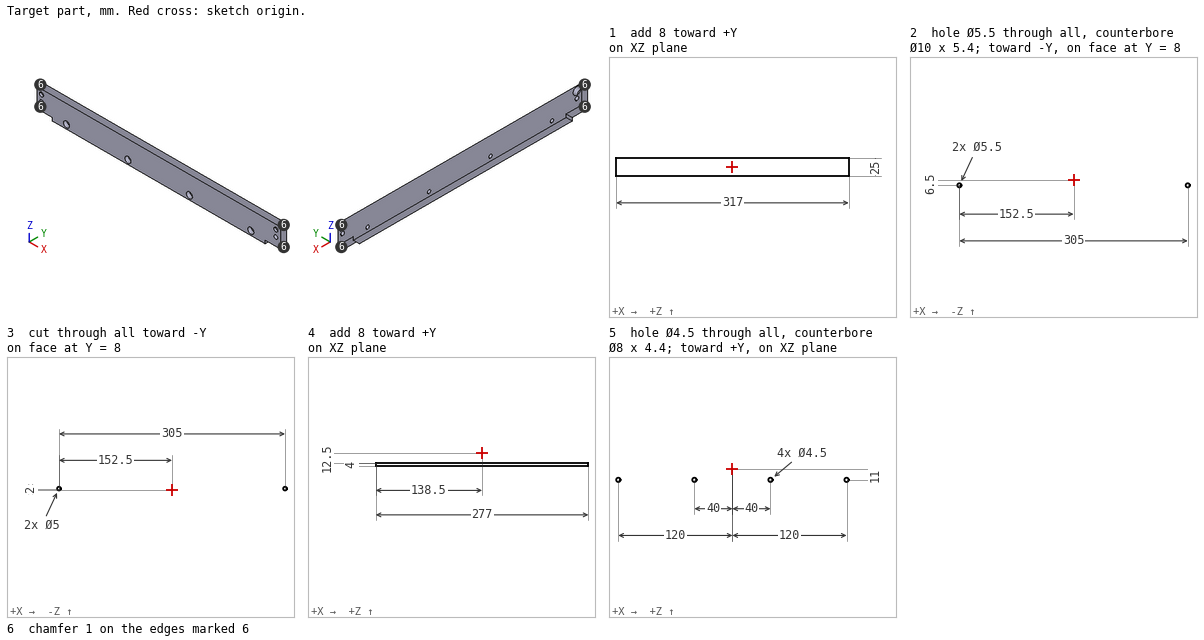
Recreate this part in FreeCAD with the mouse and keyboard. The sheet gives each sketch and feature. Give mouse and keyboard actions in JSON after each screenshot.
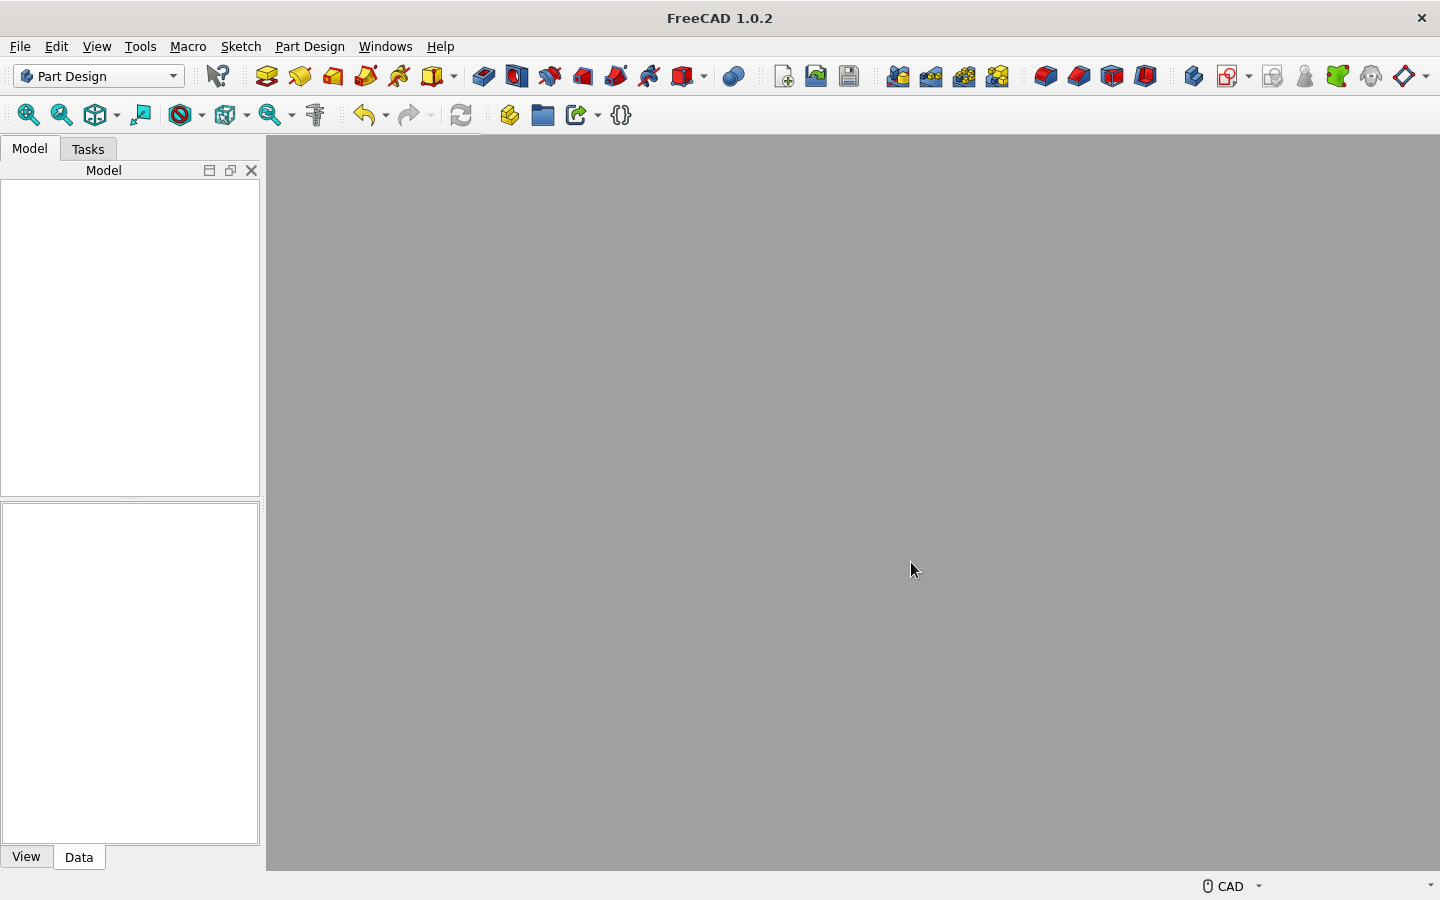
{"action": "left_click", "coordinate": [783, 76]}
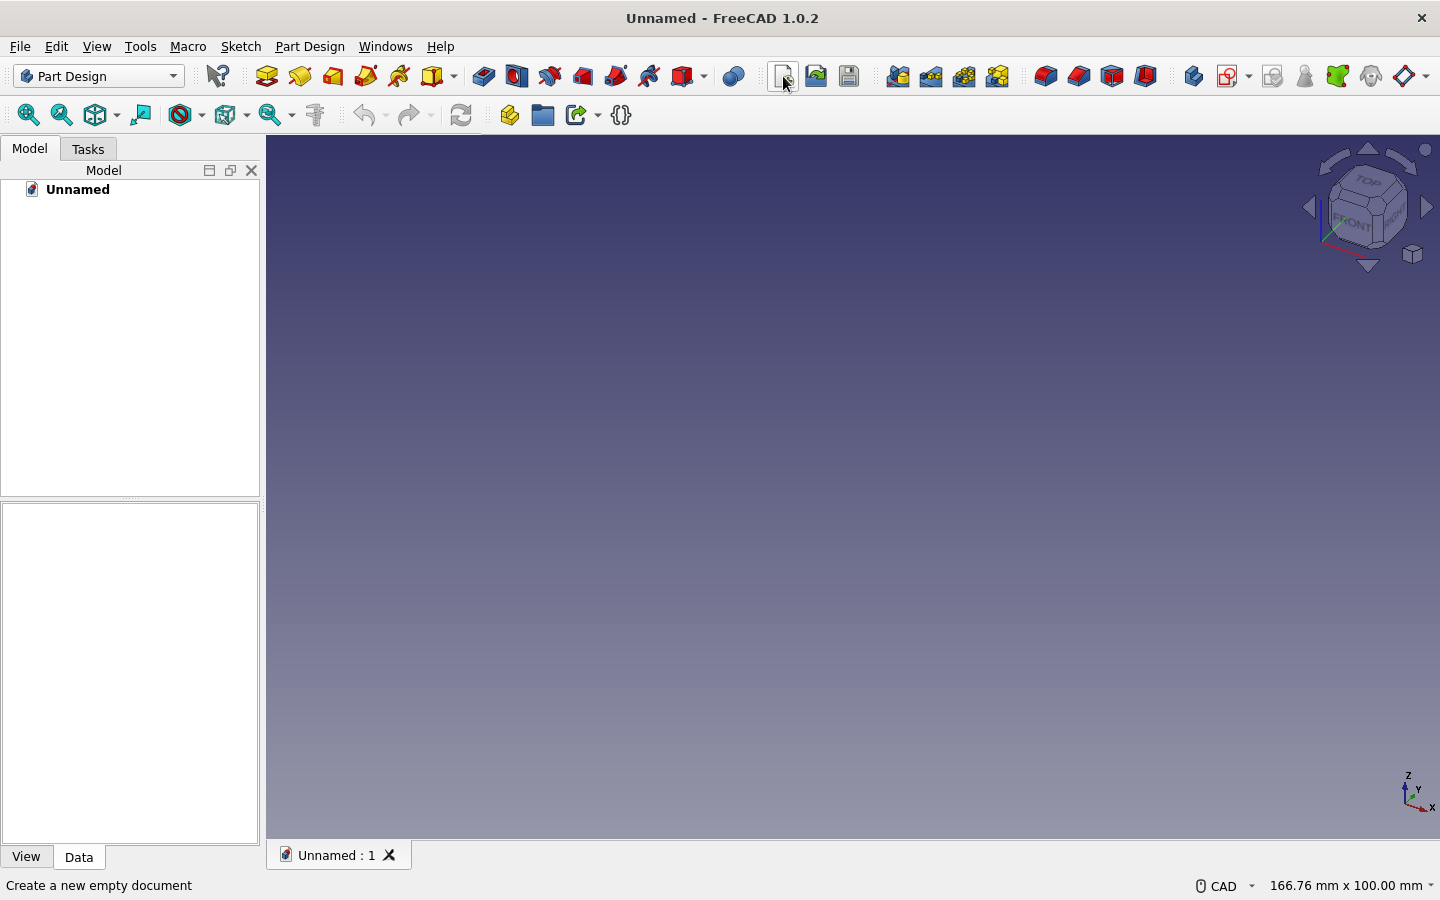
{"action": "left_click", "coordinate": [1226, 76]}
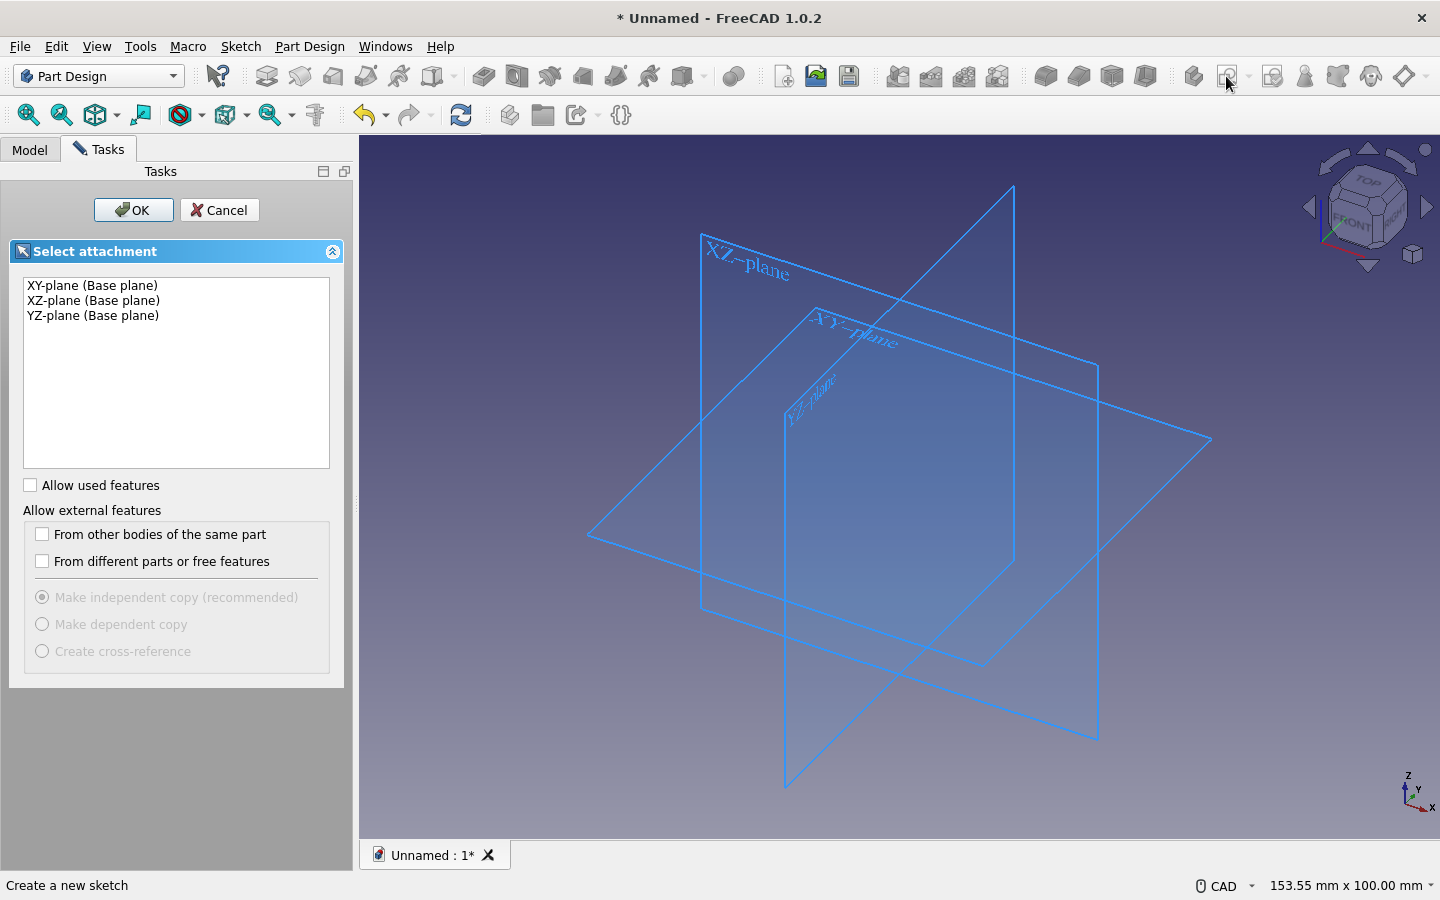
{"action": "left_click", "coordinate": [84, 300]}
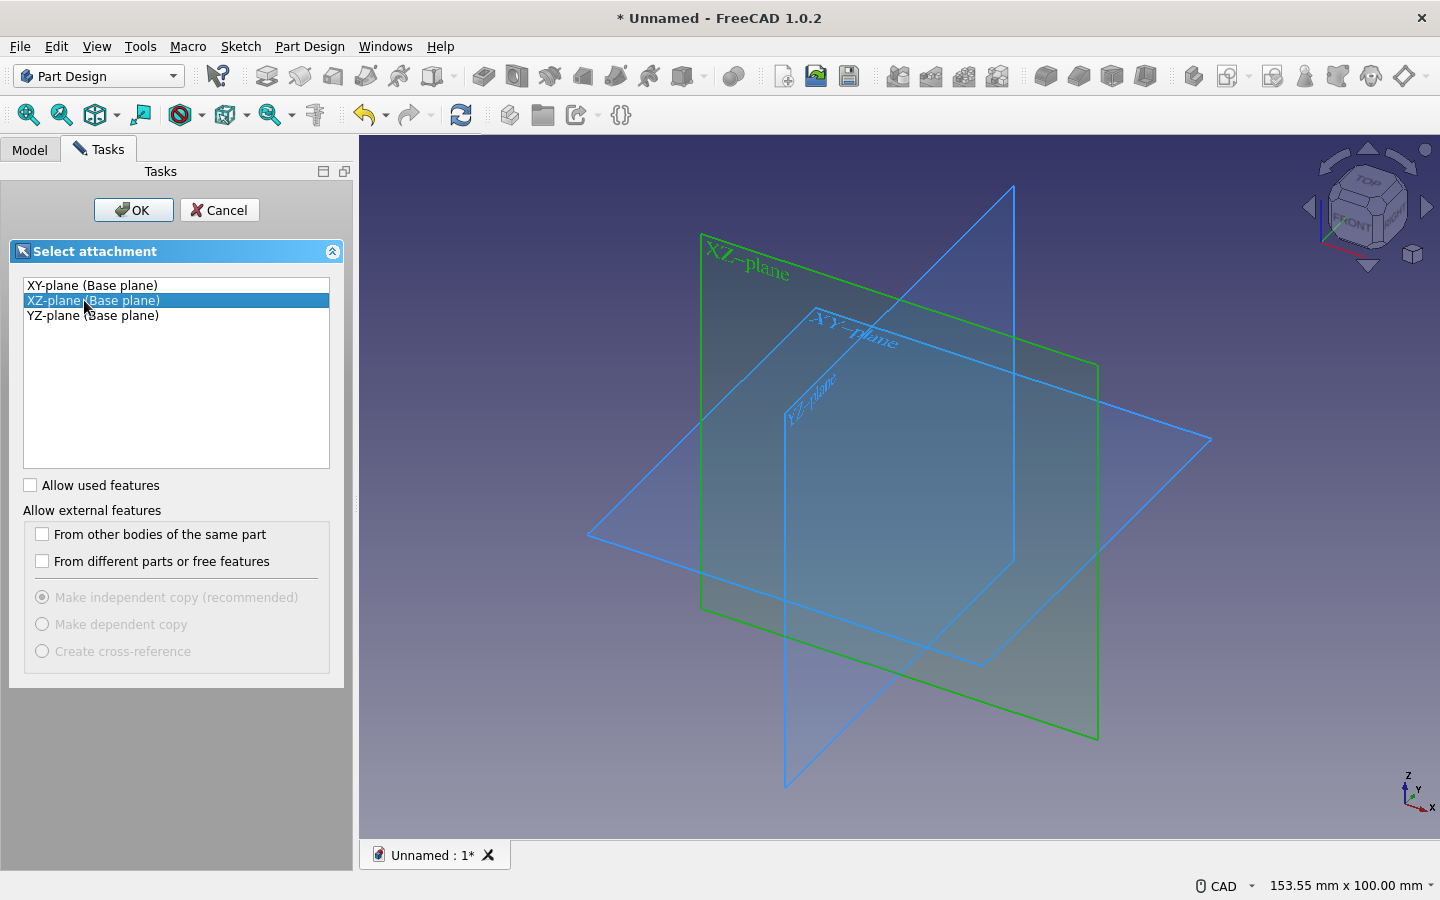
{"action": "left_click", "coordinate": [134, 210]}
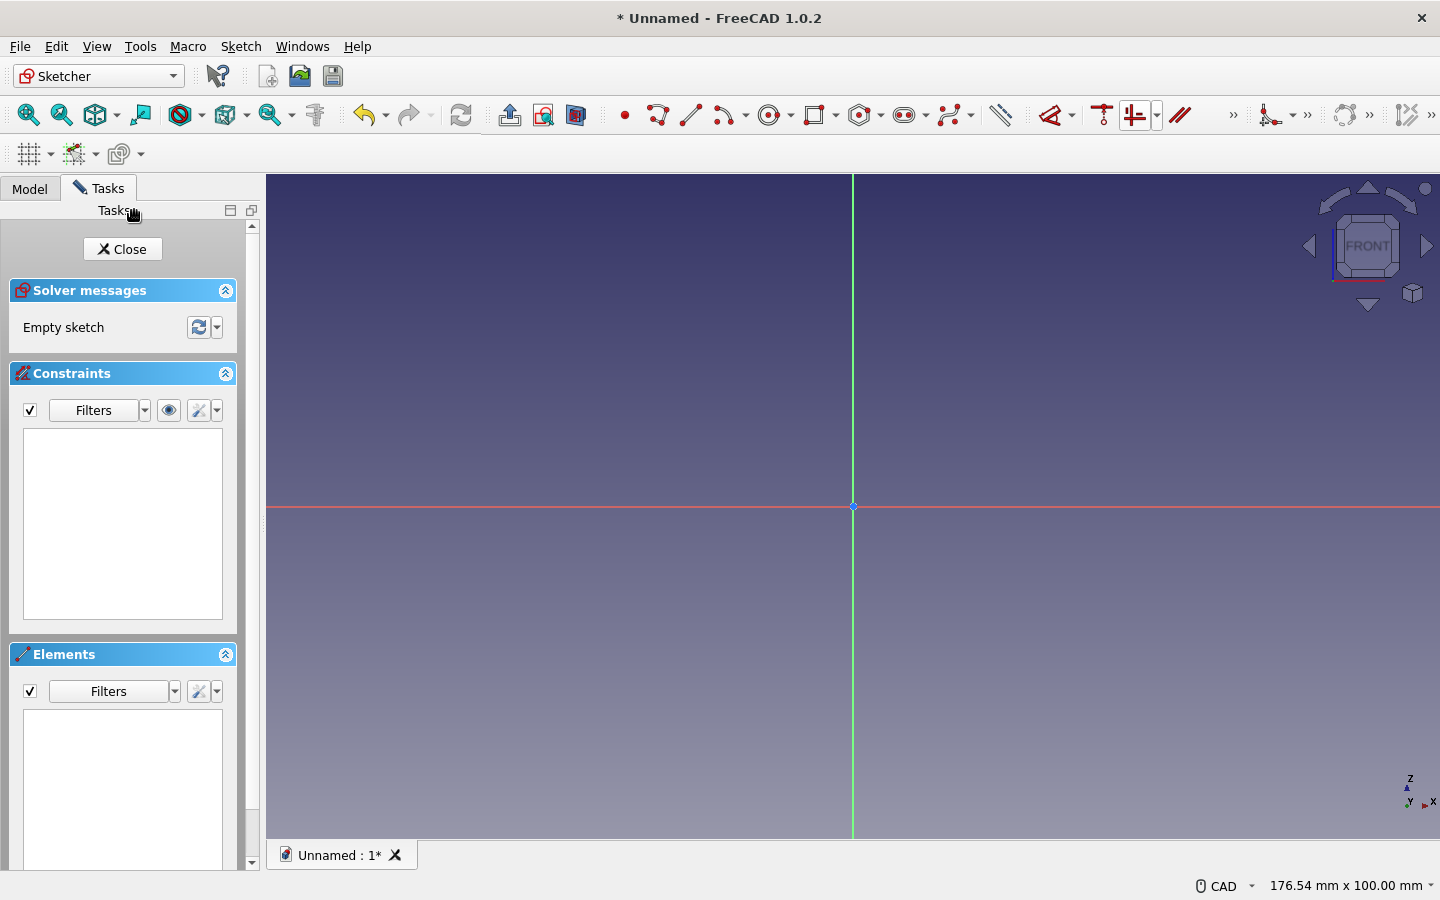
{"action": "scroll", "coordinate": [755, 506], "scroll_direction": "down", "scroll_amount": 6}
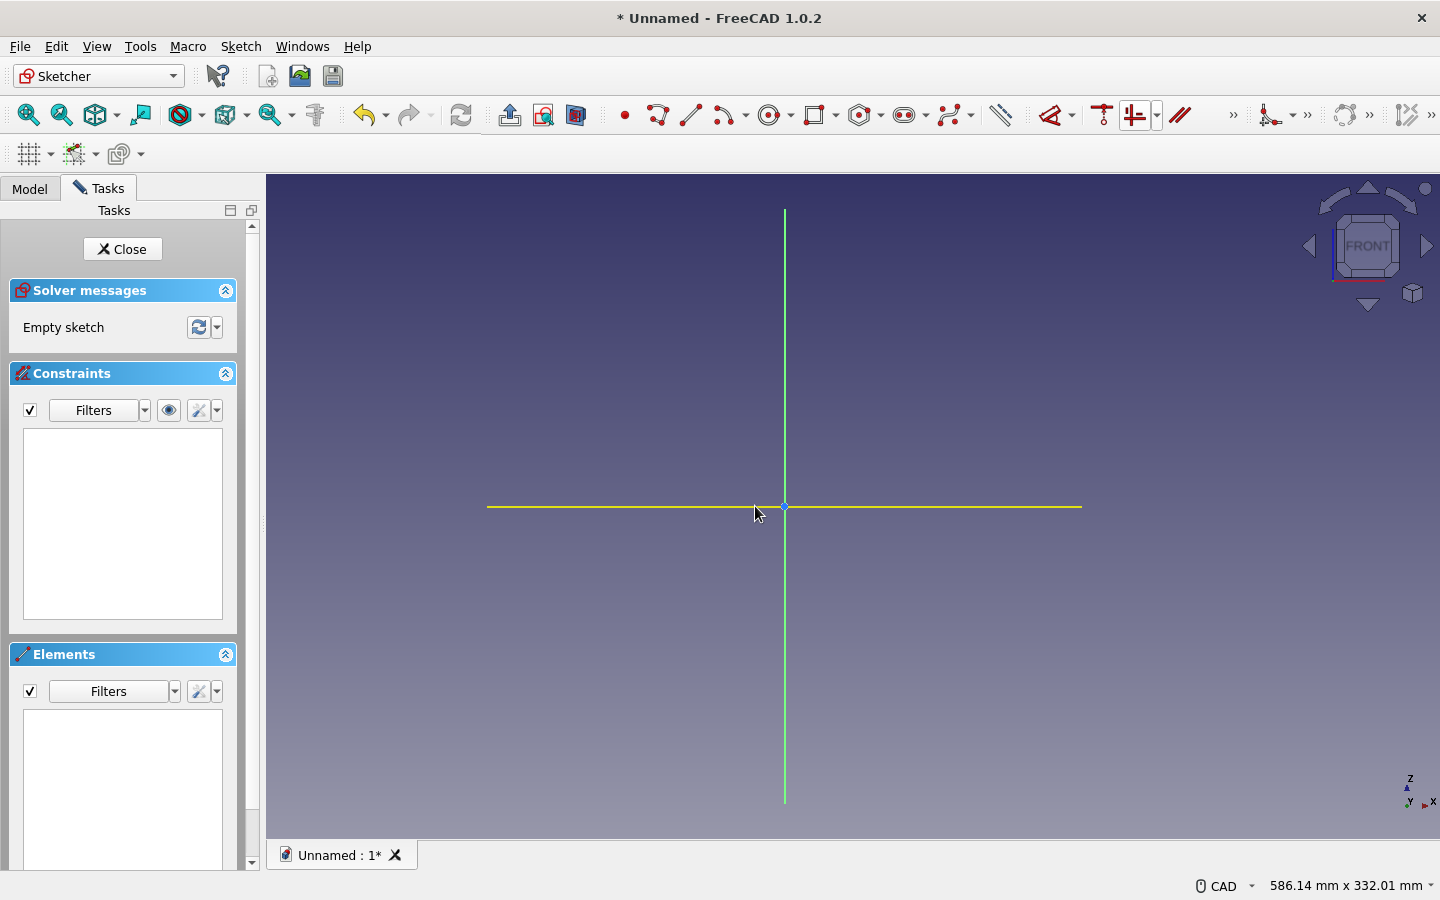
{"action": "left_click", "coordinate": [836, 116]}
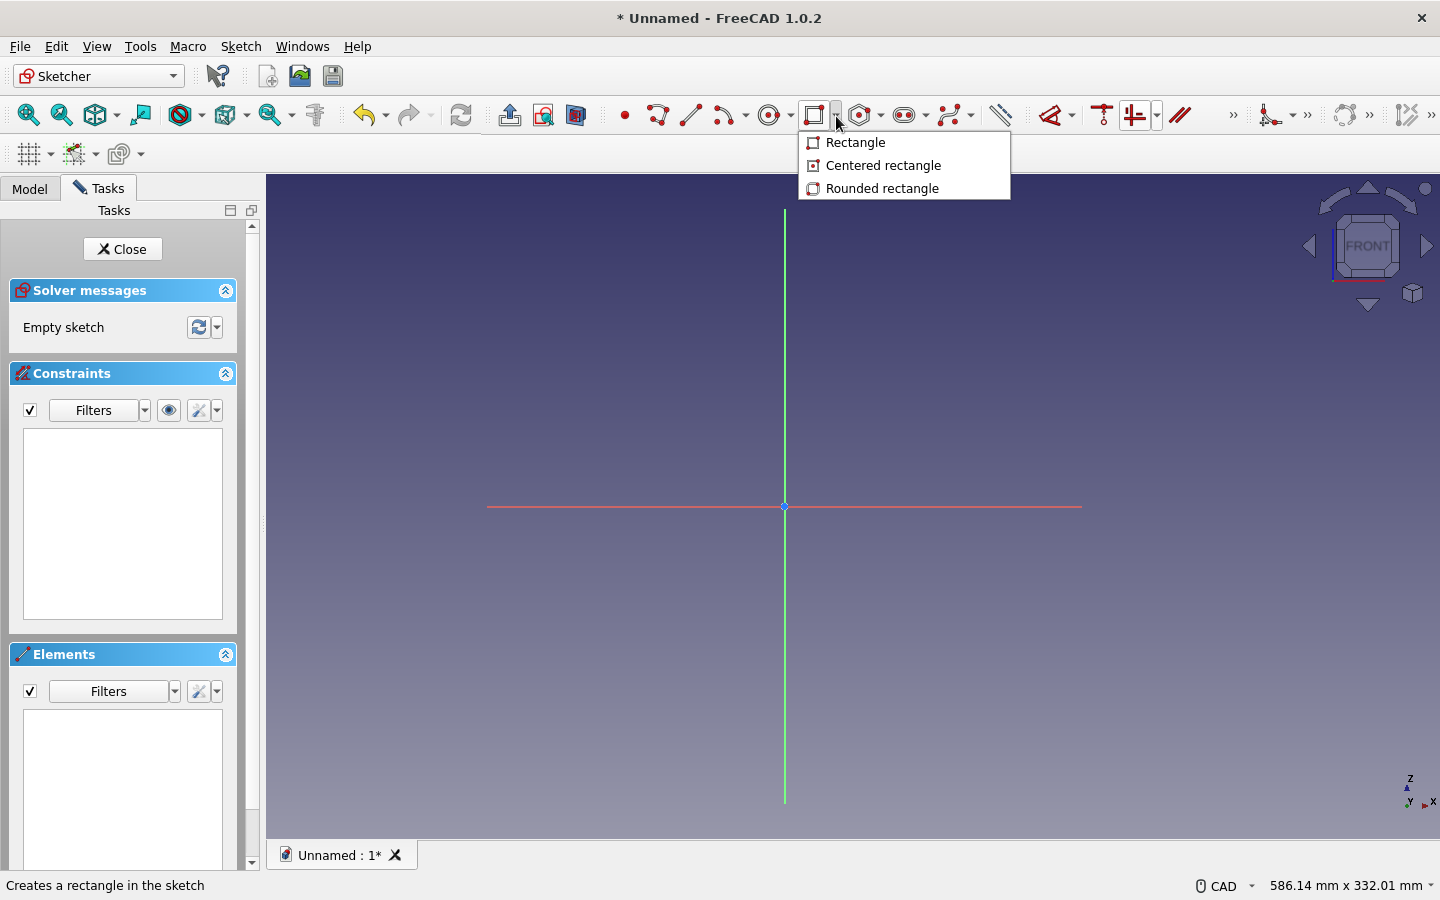
{"action": "left_click", "coordinate": [904, 166]}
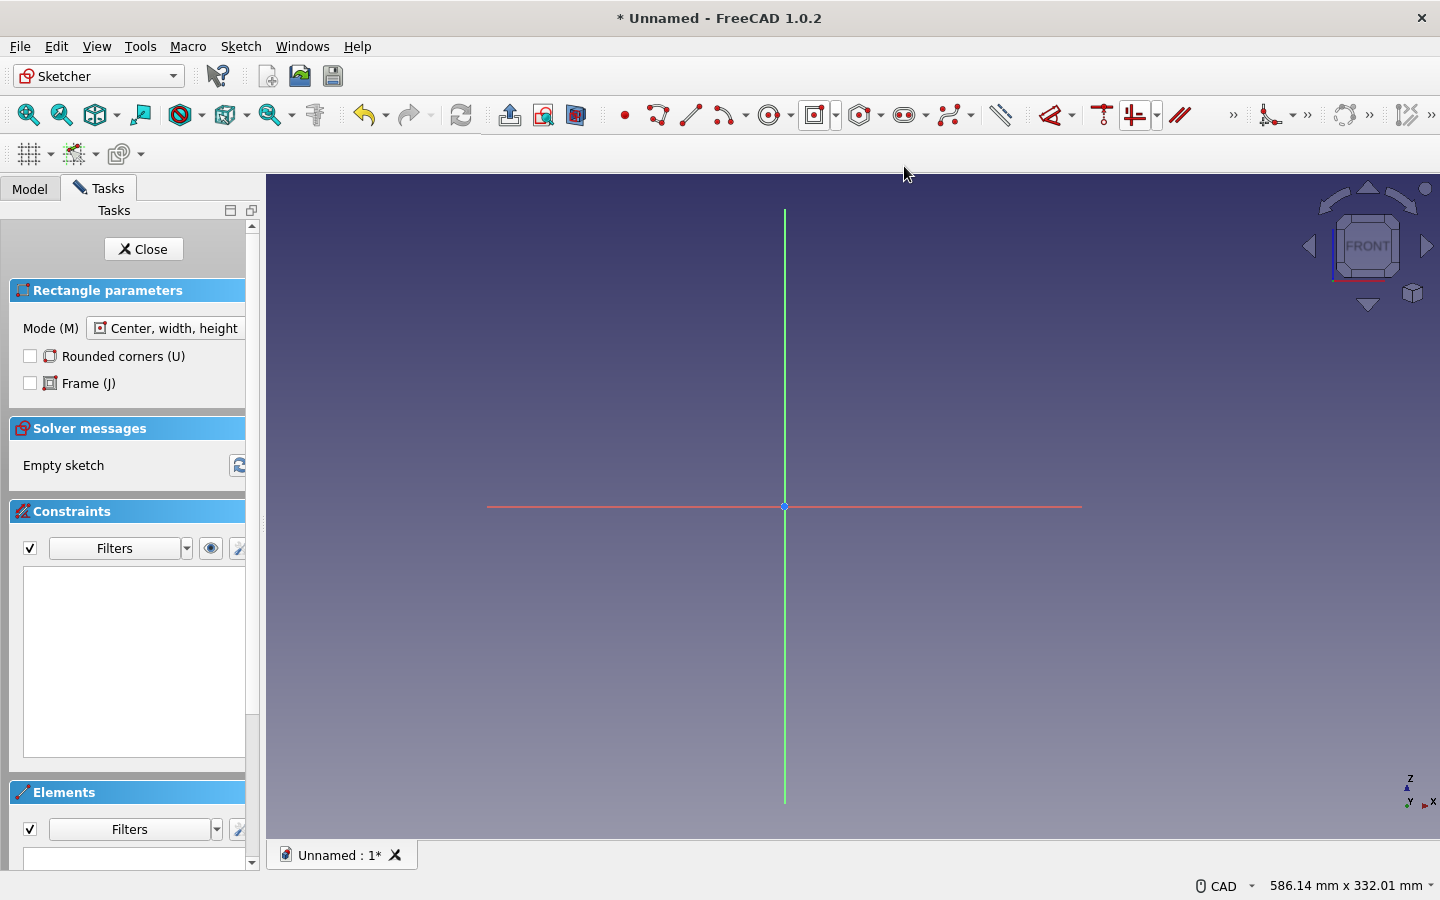
{"action": "left_click", "coordinate": [785, 506]}
{"action": "mouse_move", "coordinate": [1102, 481]}